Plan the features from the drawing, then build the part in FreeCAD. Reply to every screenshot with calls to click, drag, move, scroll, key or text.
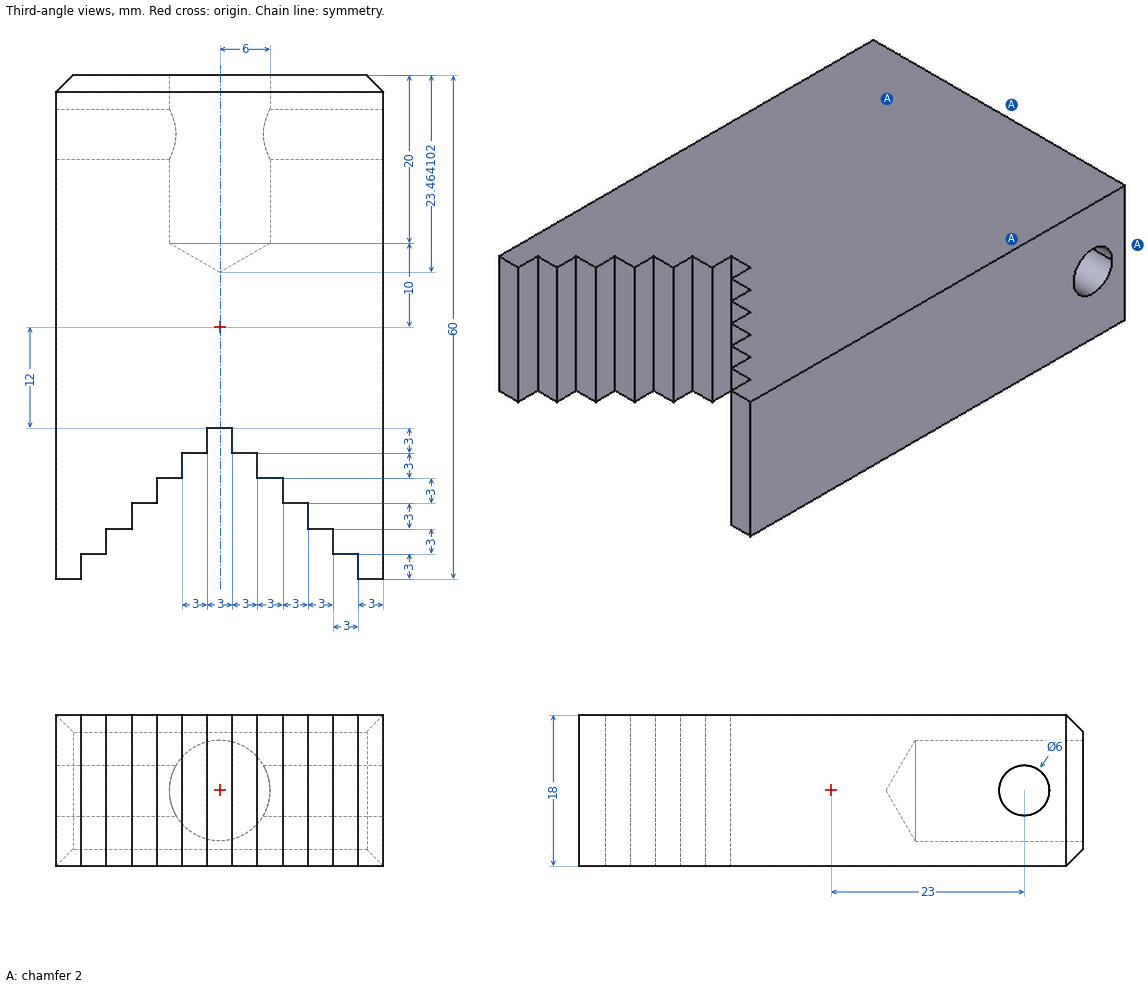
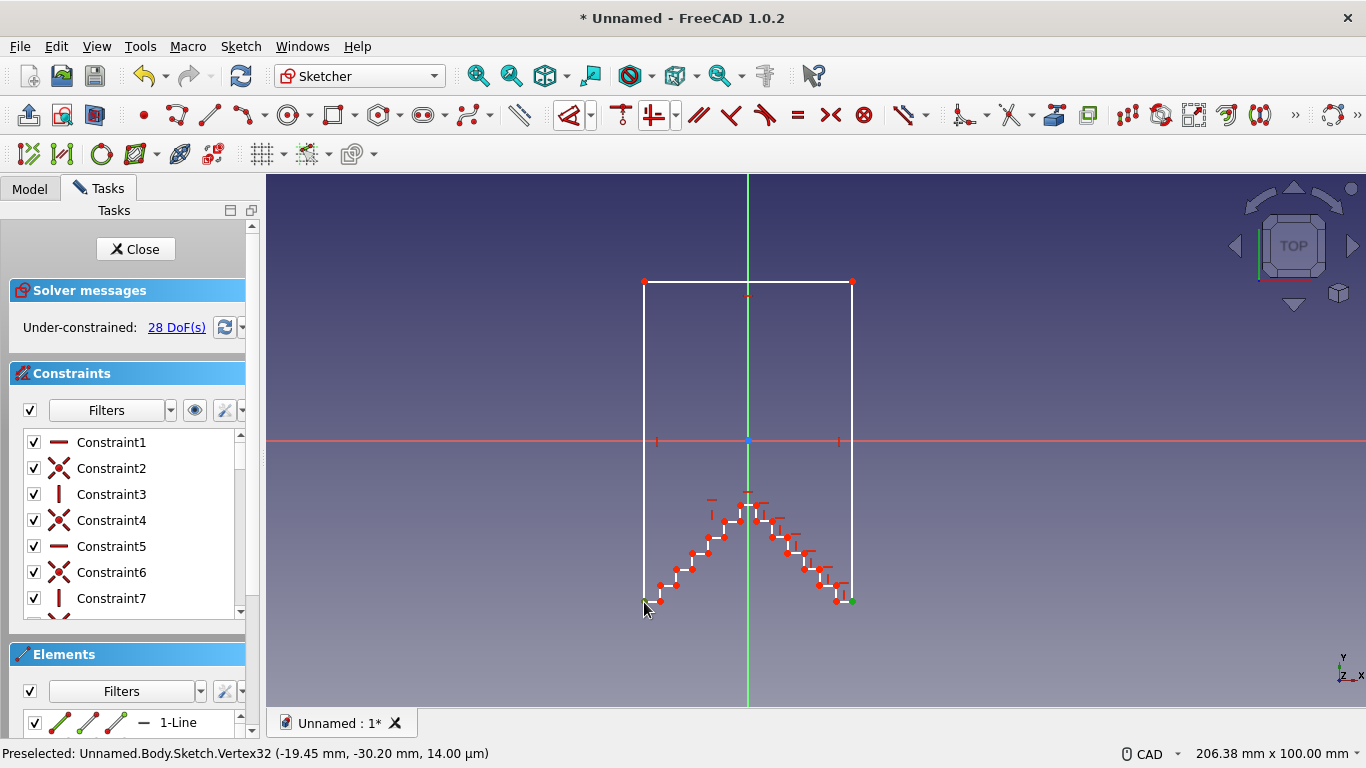
click(748, 645)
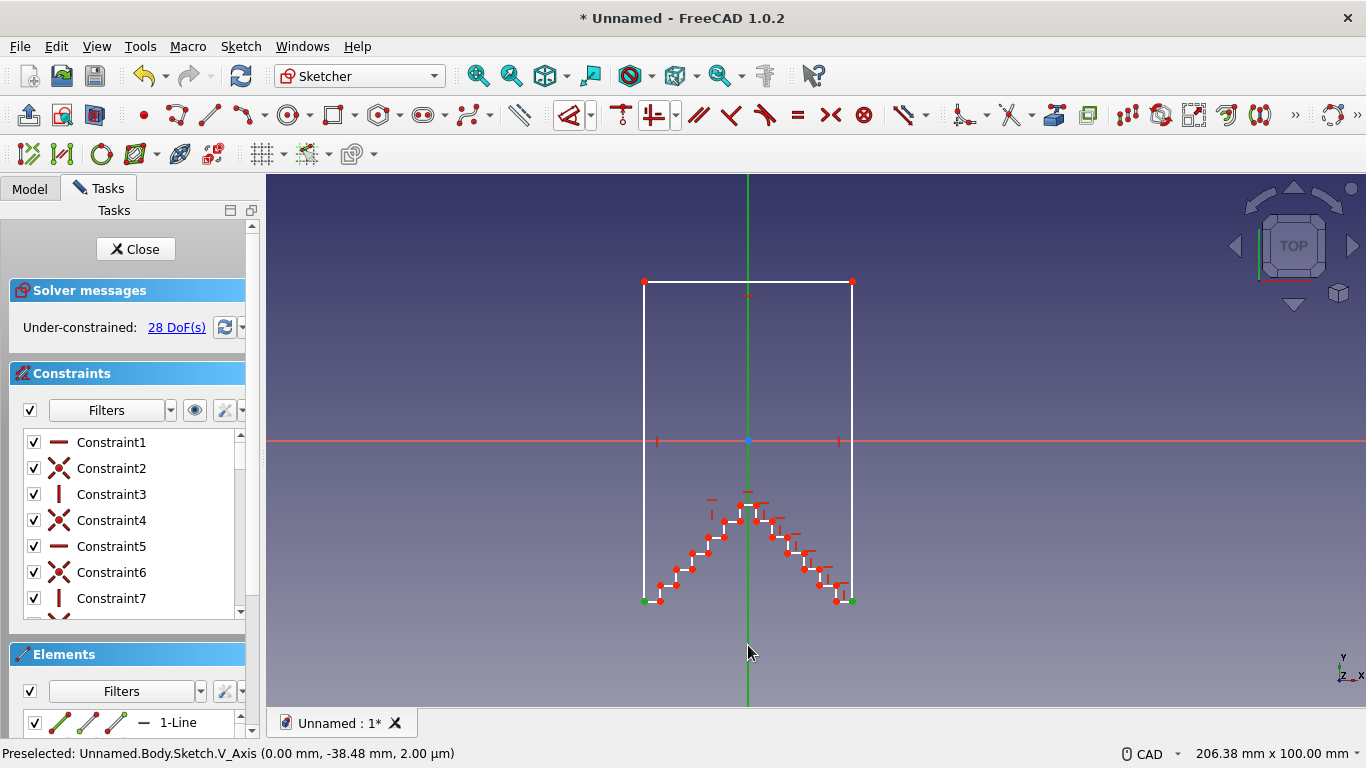
click(831, 116)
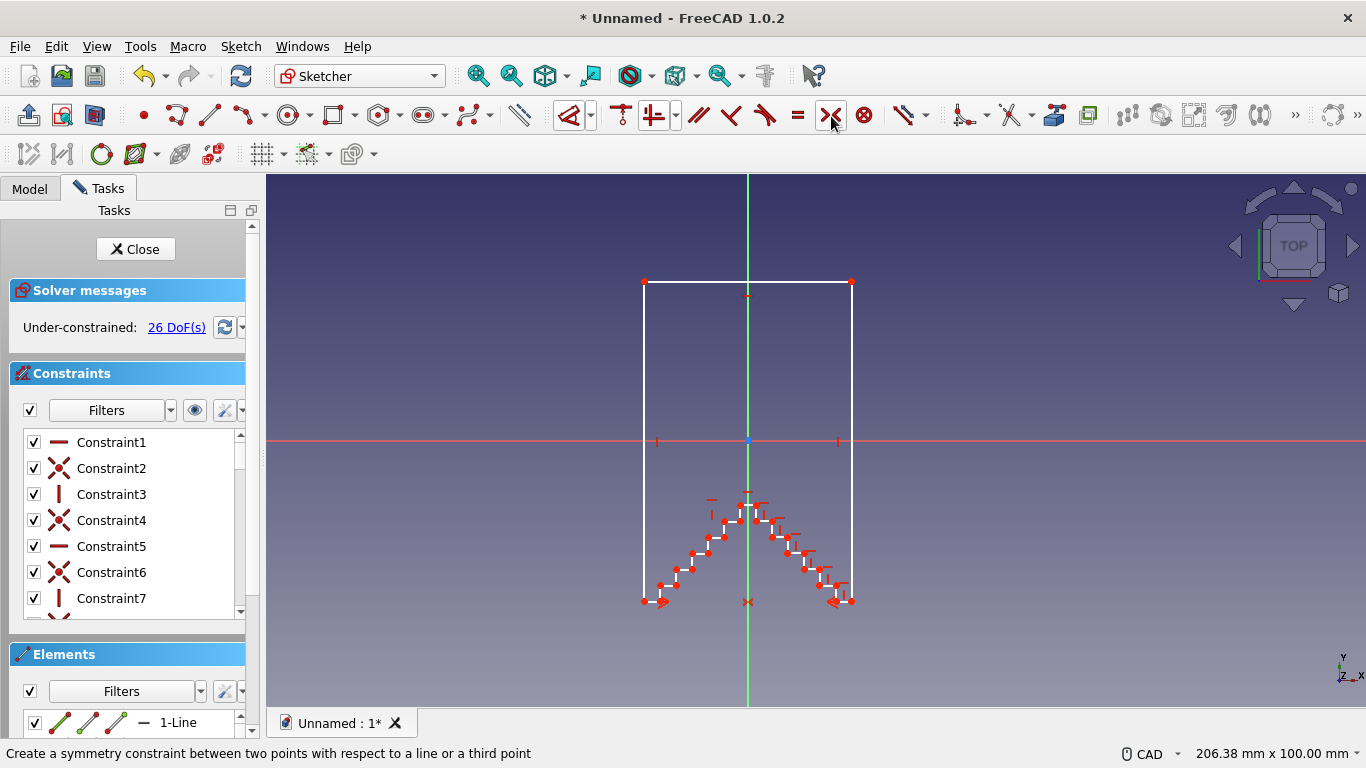
click(836, 586)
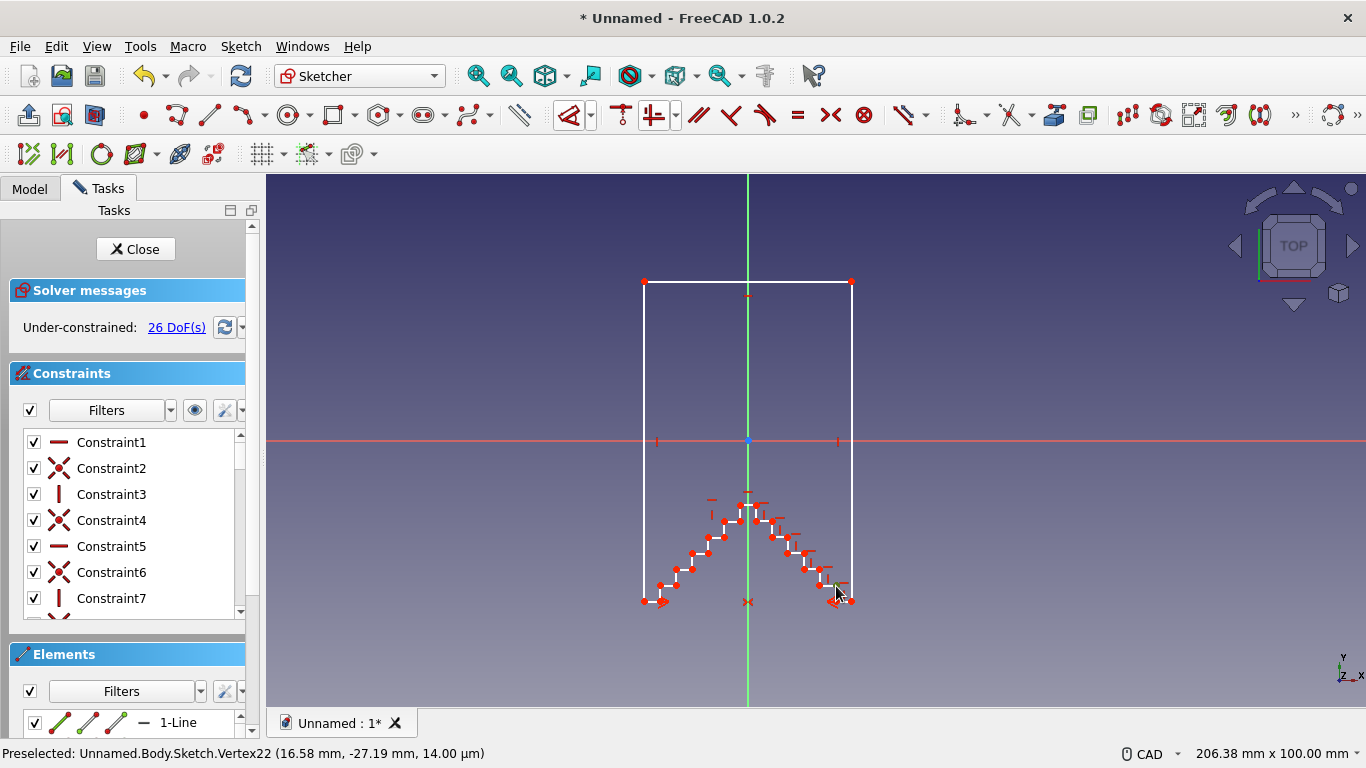
click(660, 586)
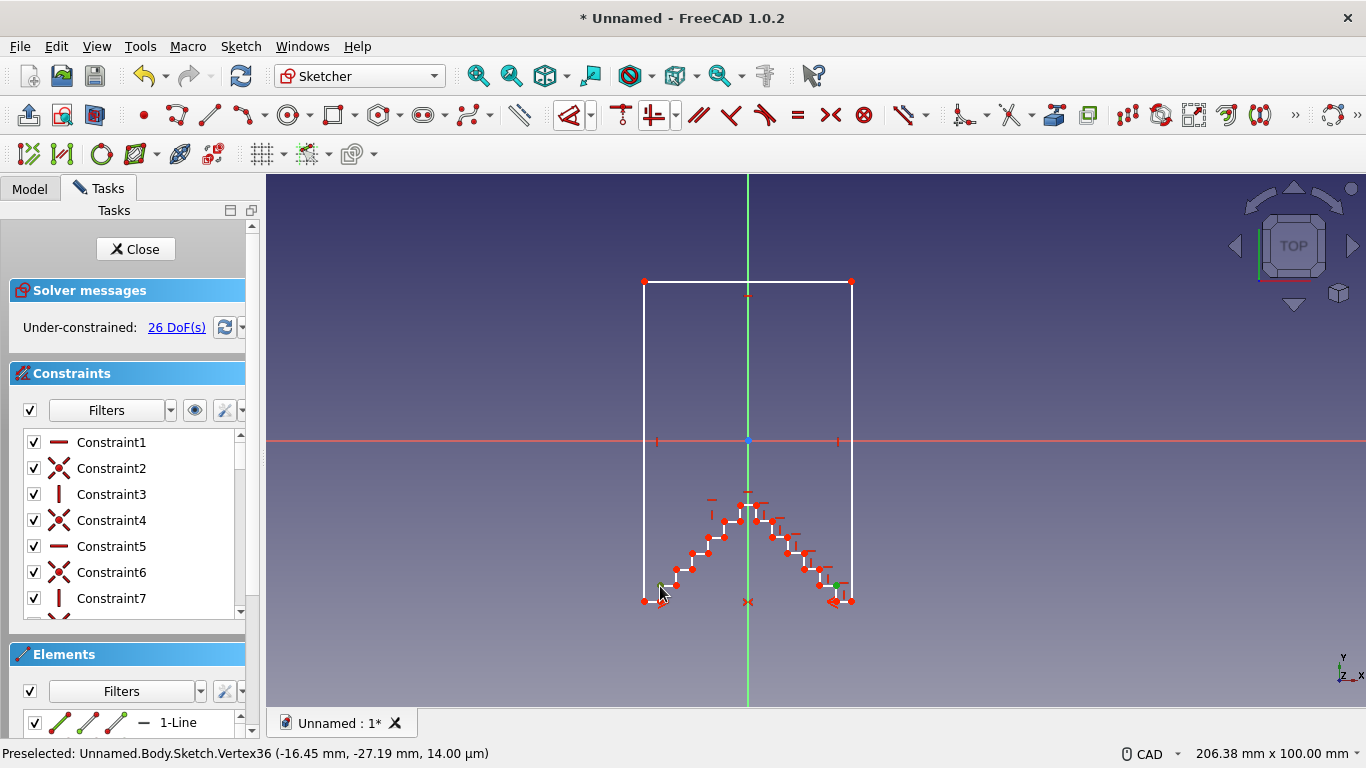
click(748, 645)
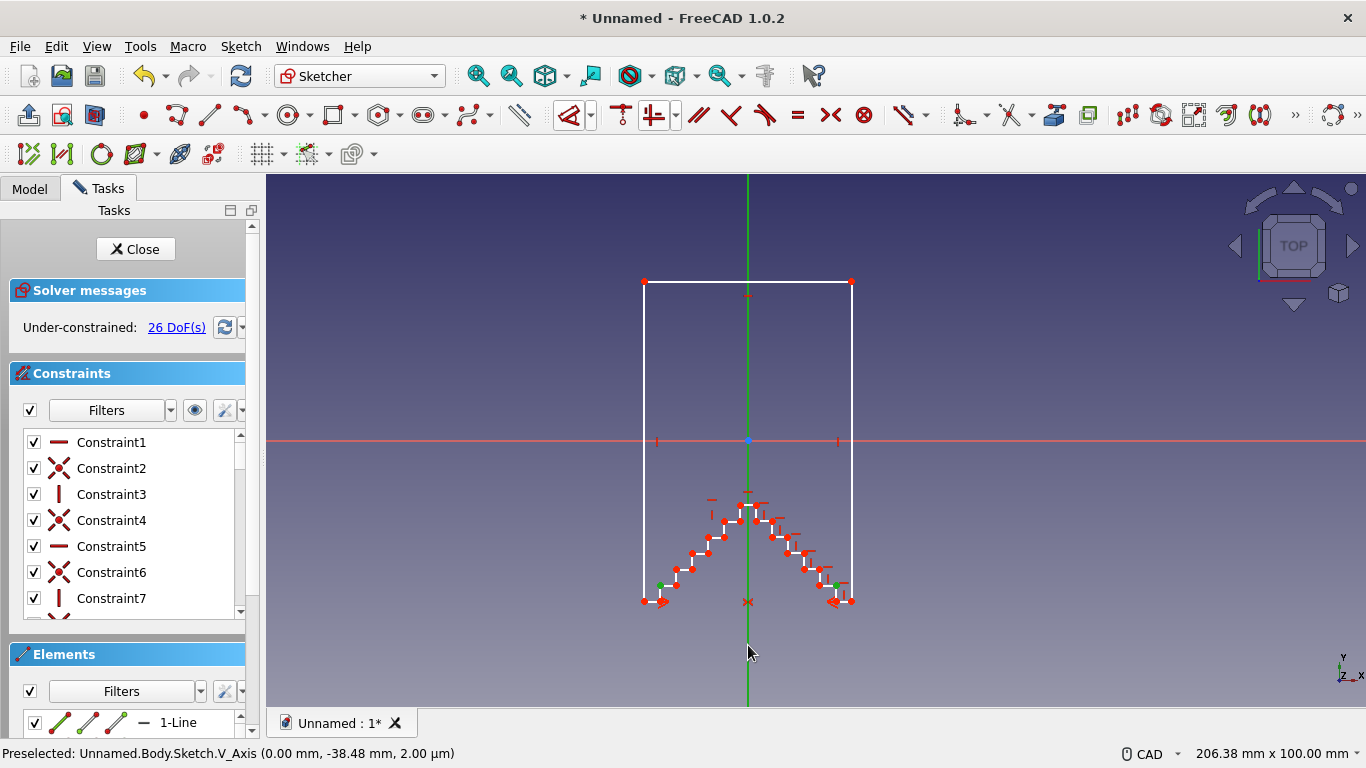
click(831, 116)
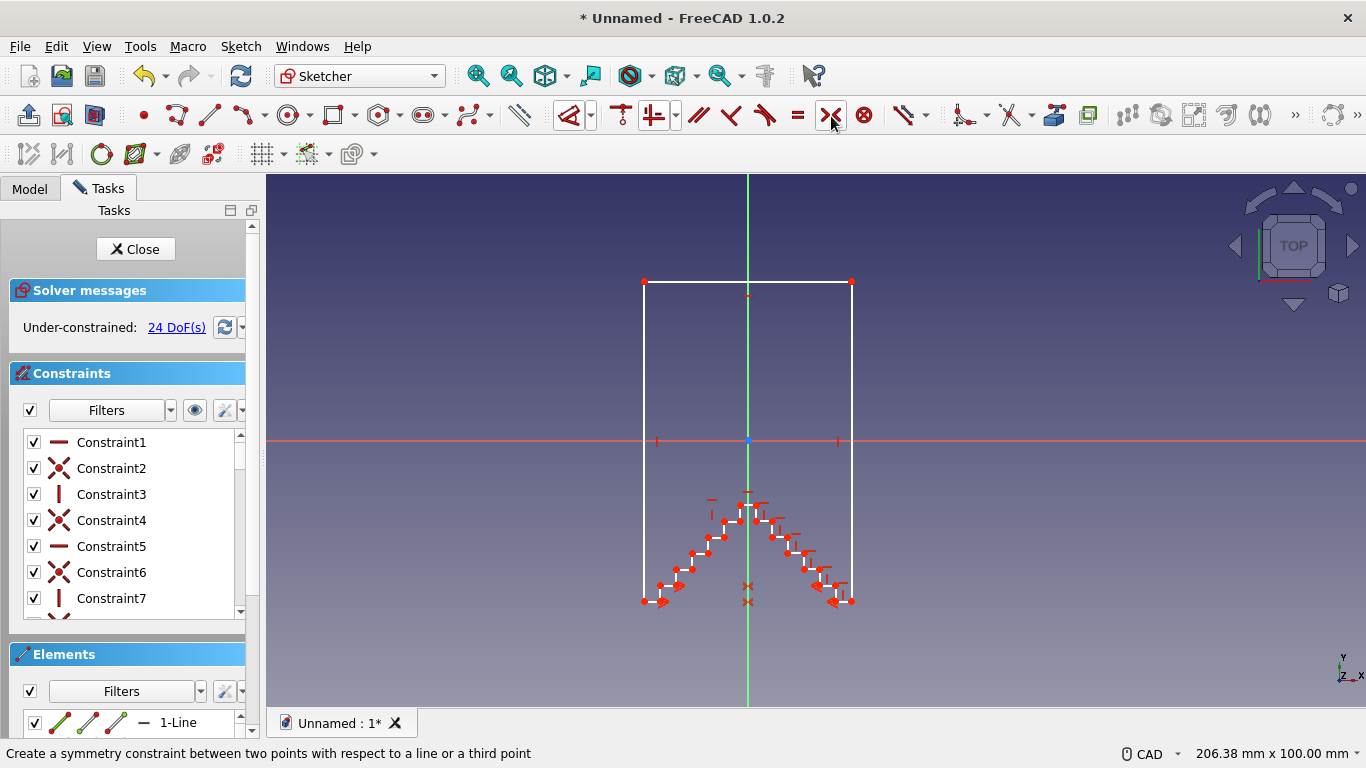
click(820, 569)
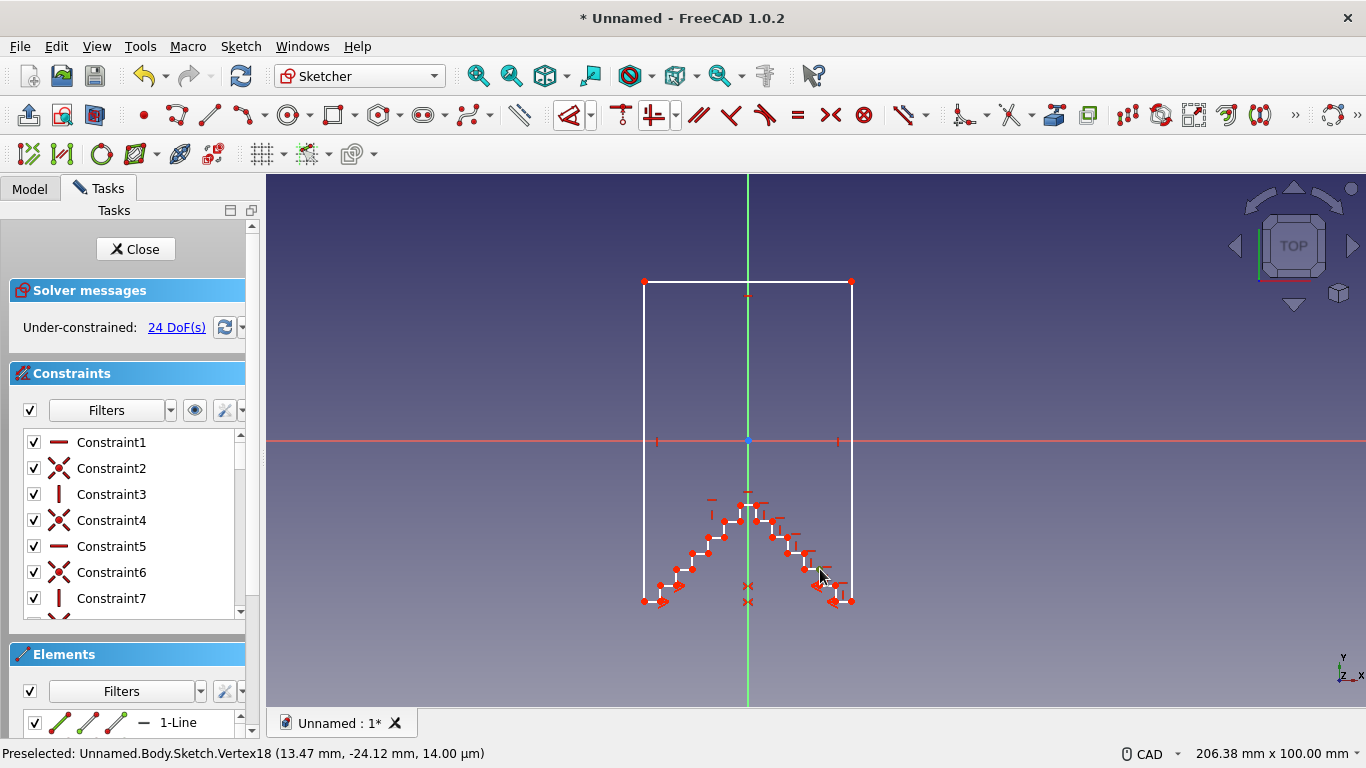
click(676, 570)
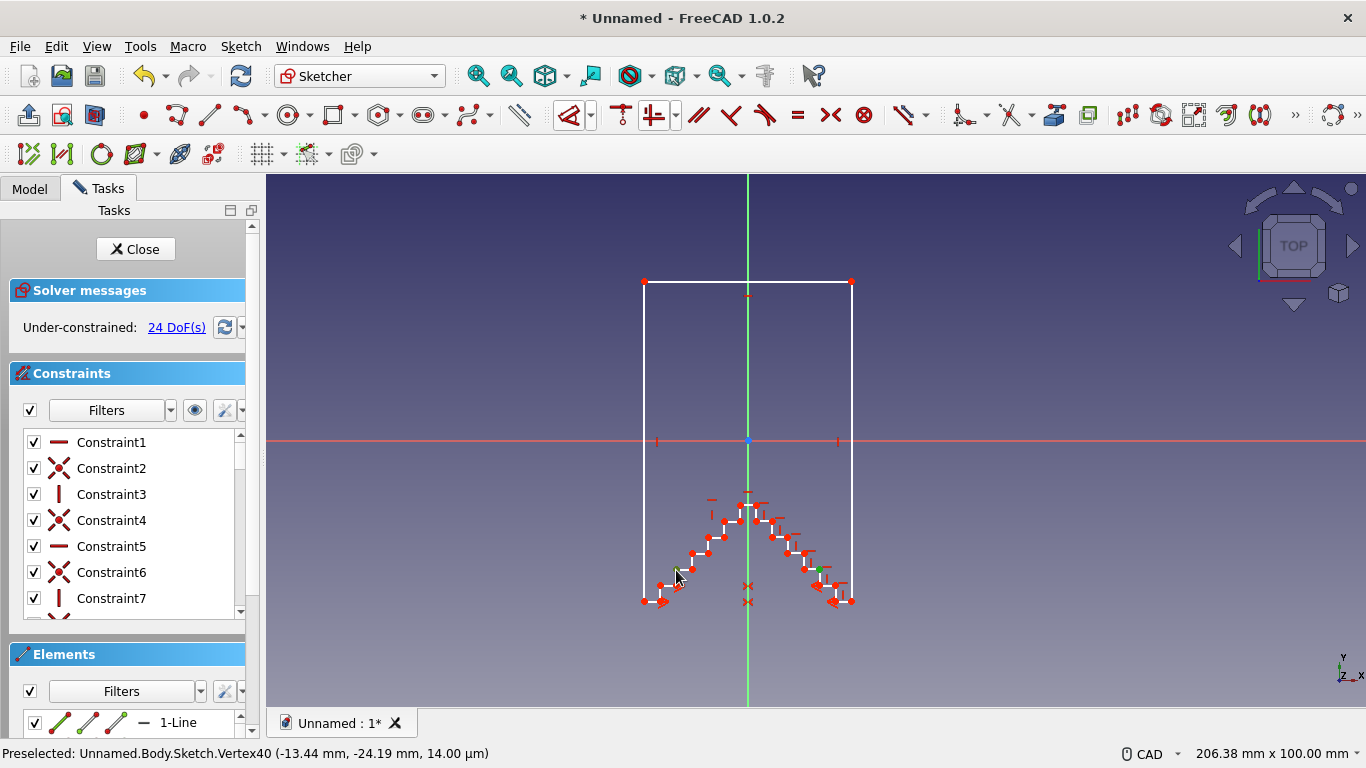
click(748, 645)